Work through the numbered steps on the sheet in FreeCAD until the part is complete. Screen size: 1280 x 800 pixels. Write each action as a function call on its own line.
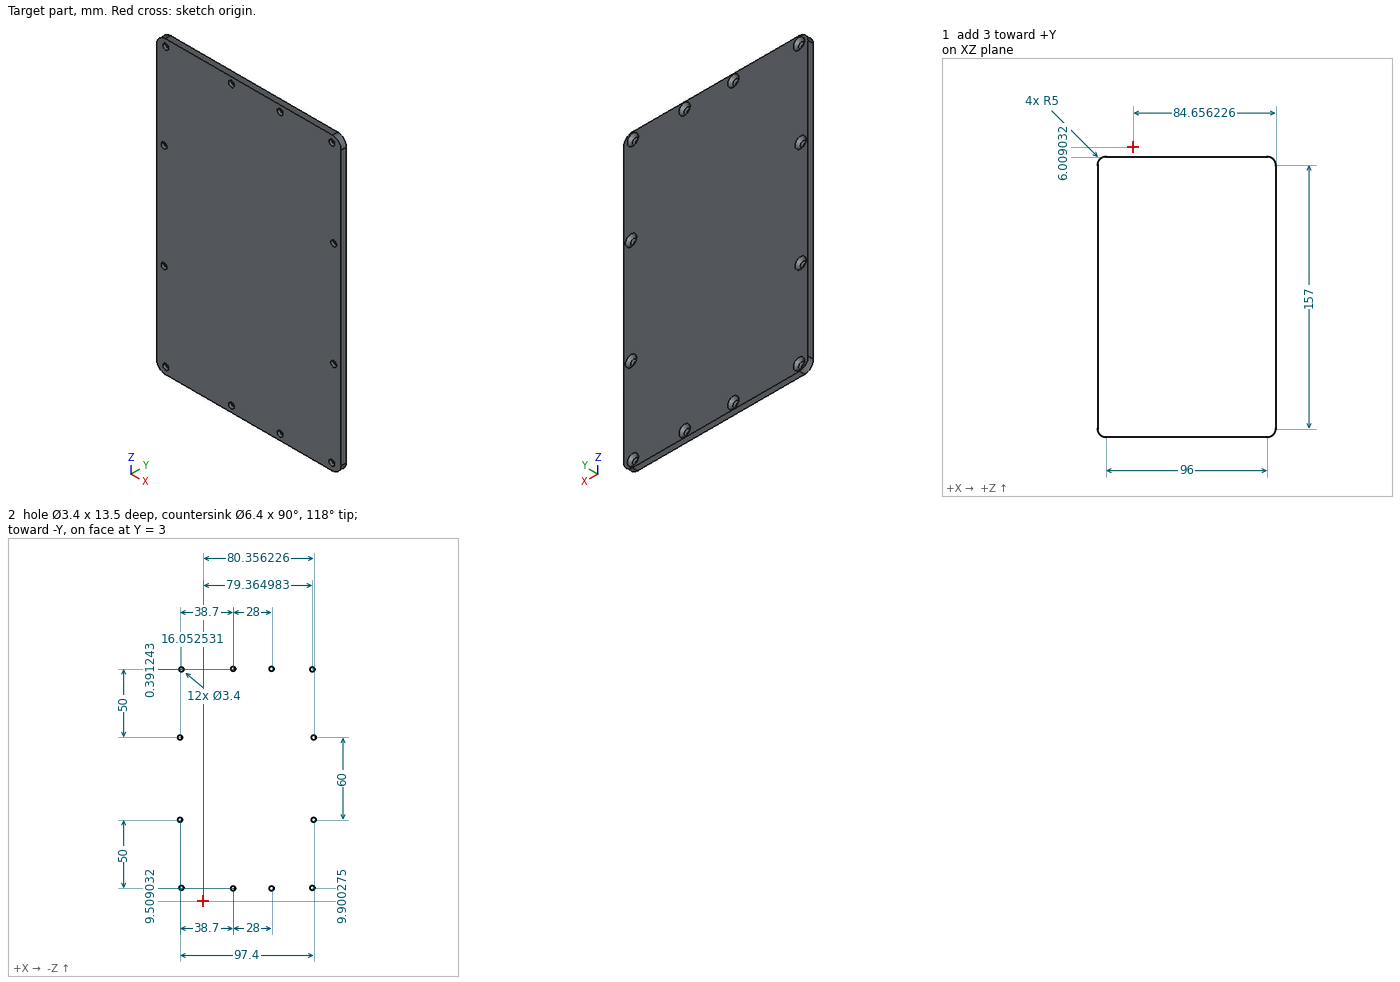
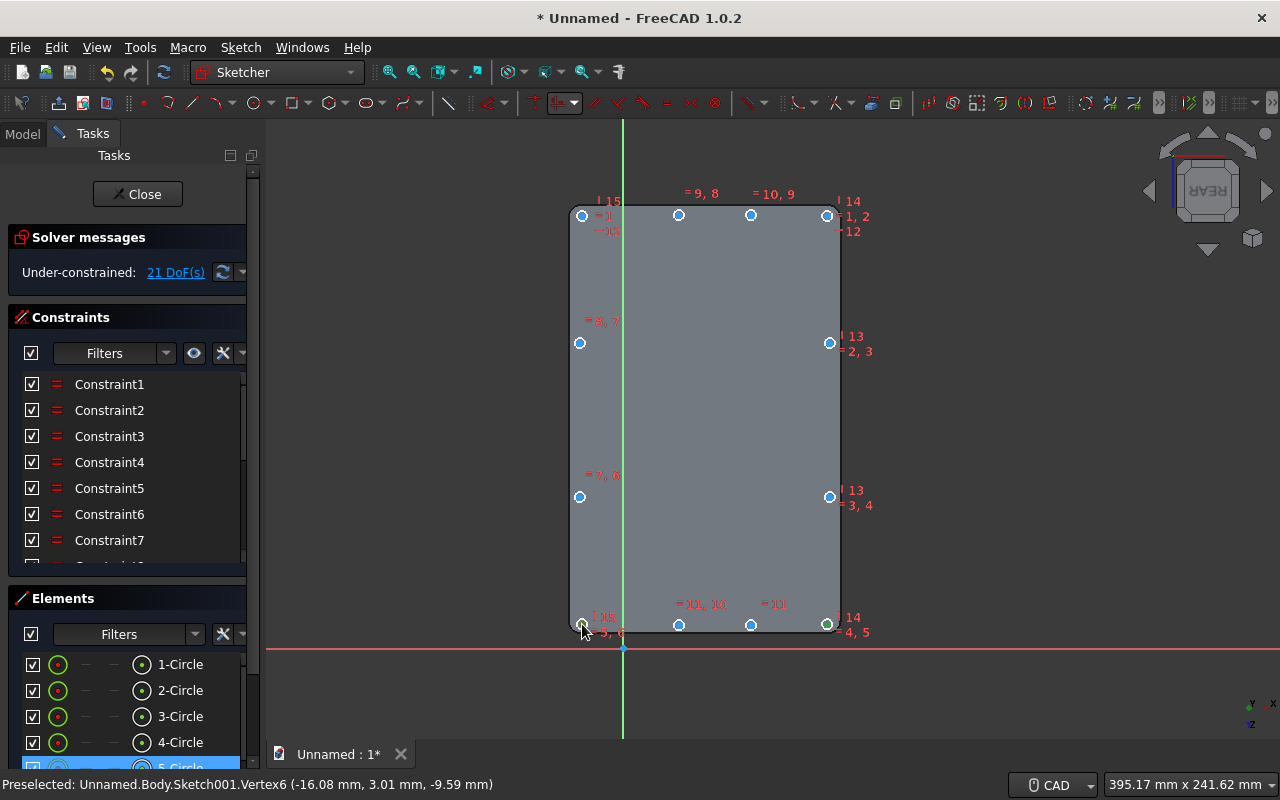
click(576, 104)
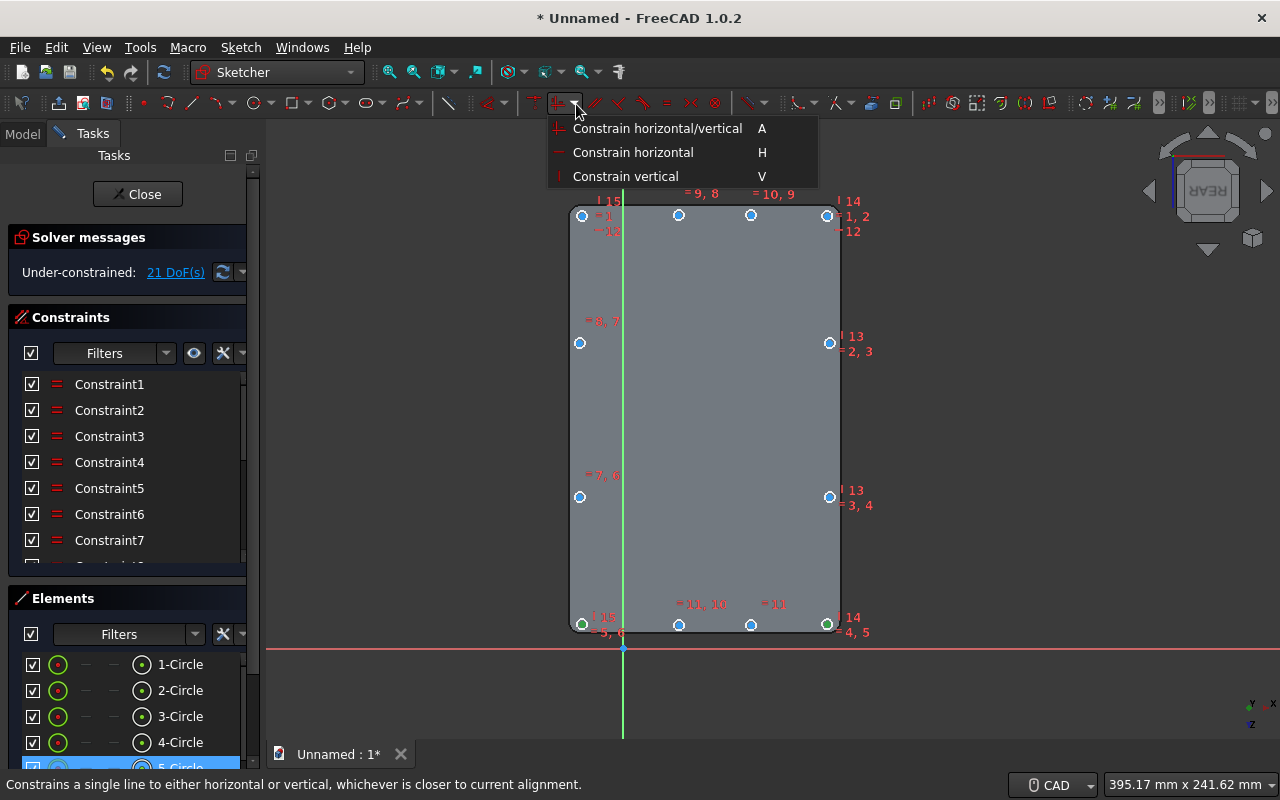
click(683, 152)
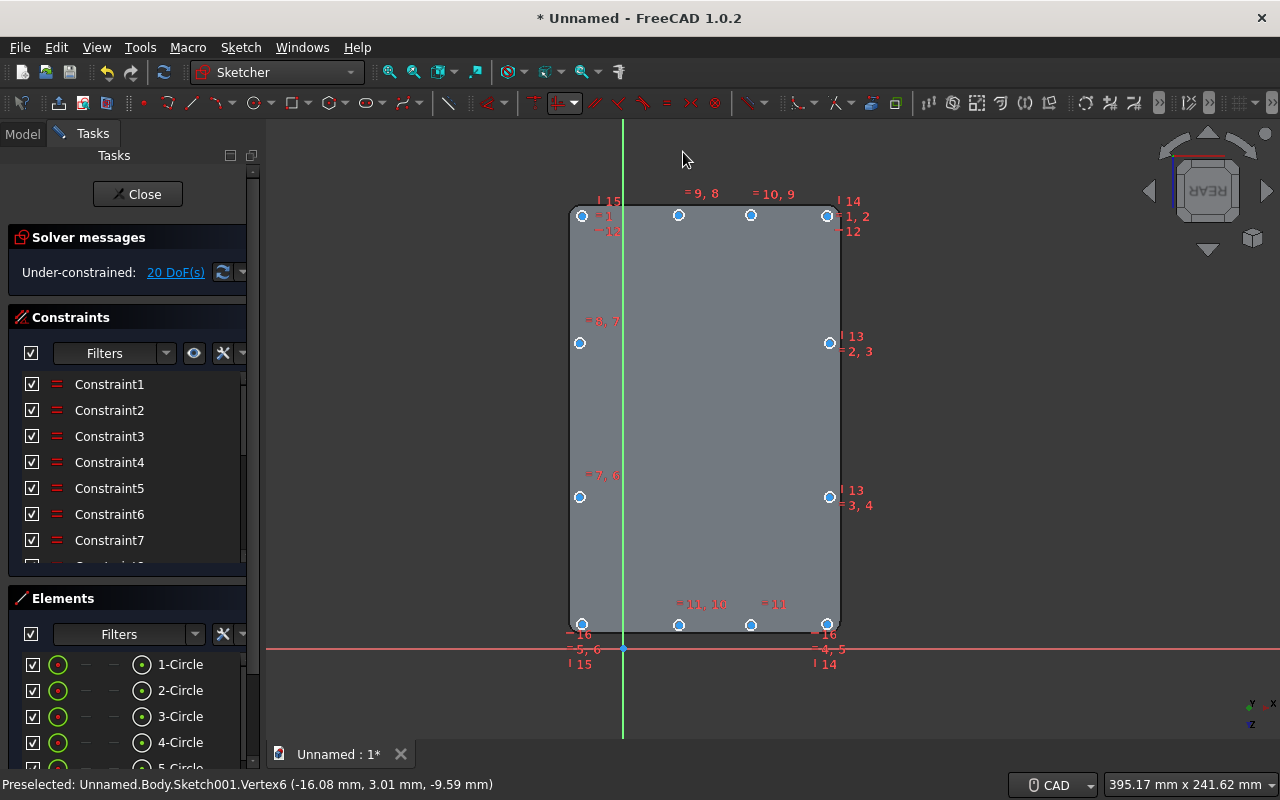
click(830, 497)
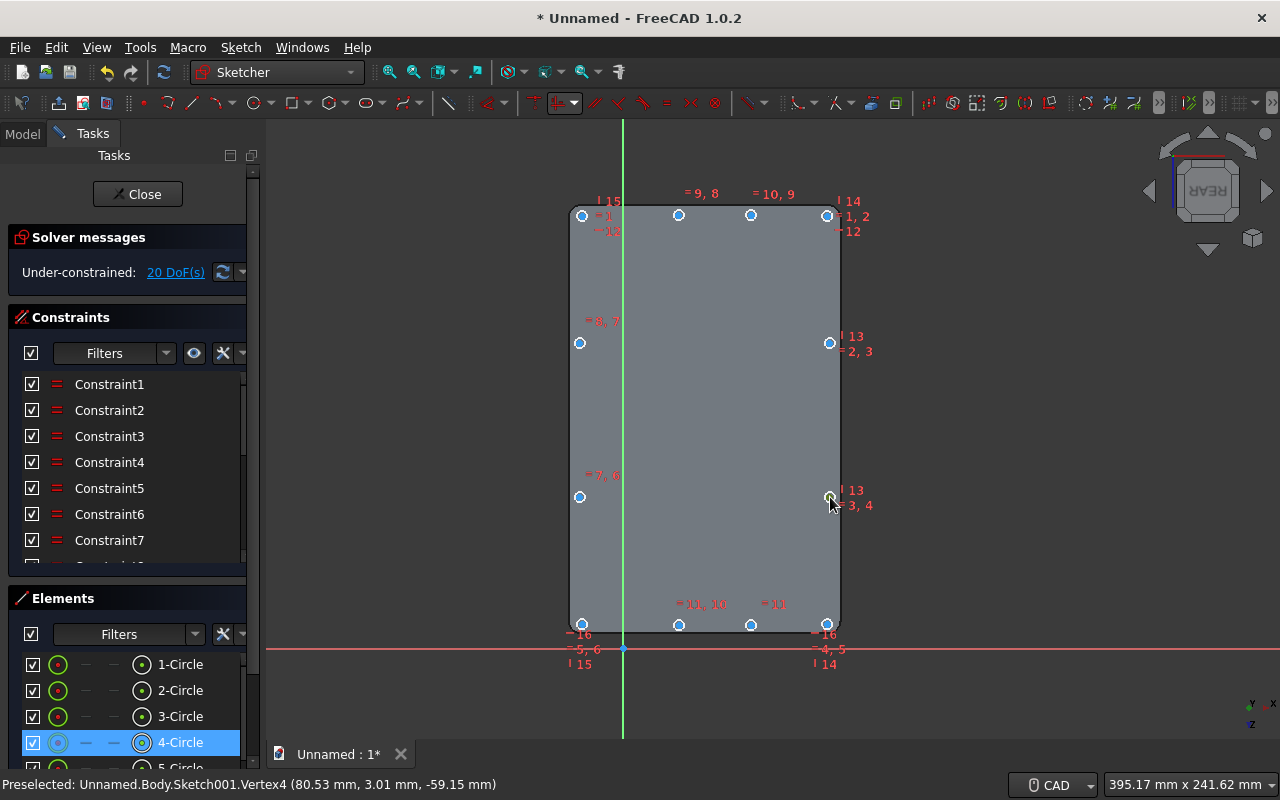
click(580, 497)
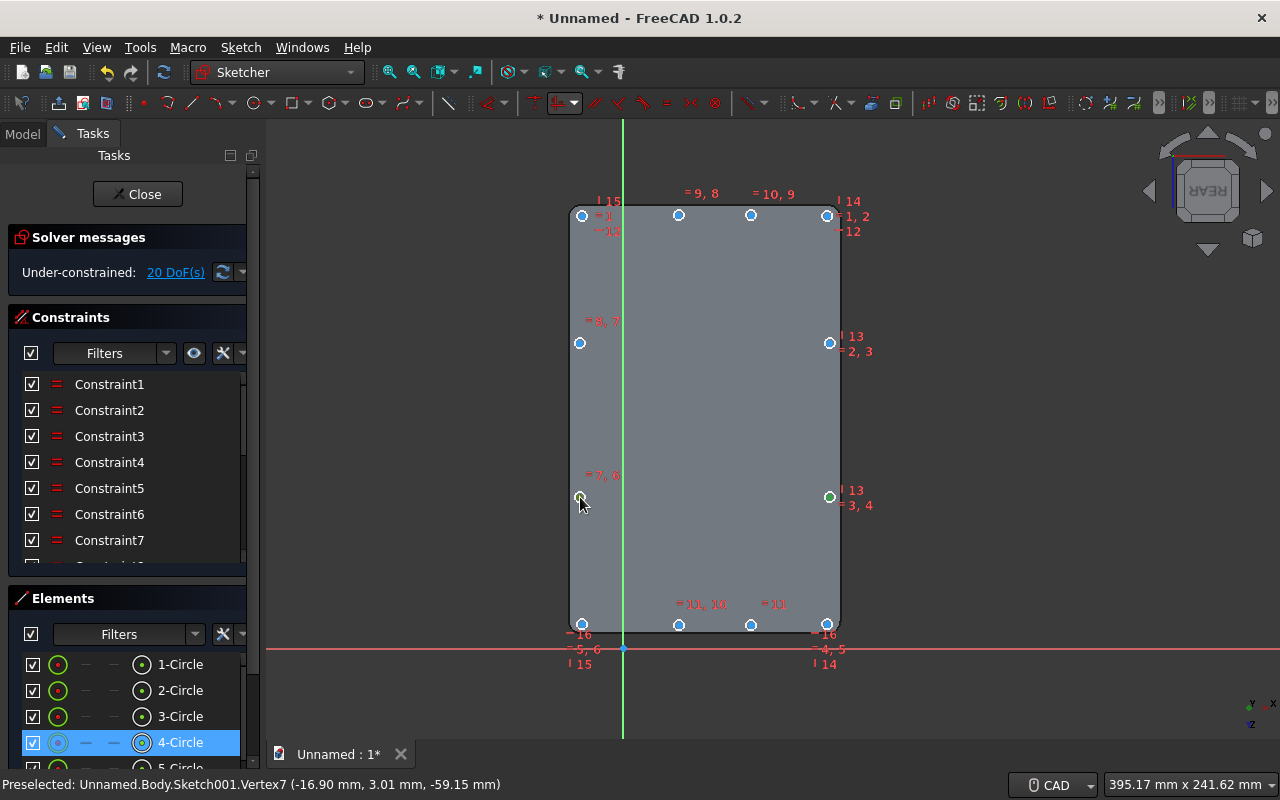
key(h)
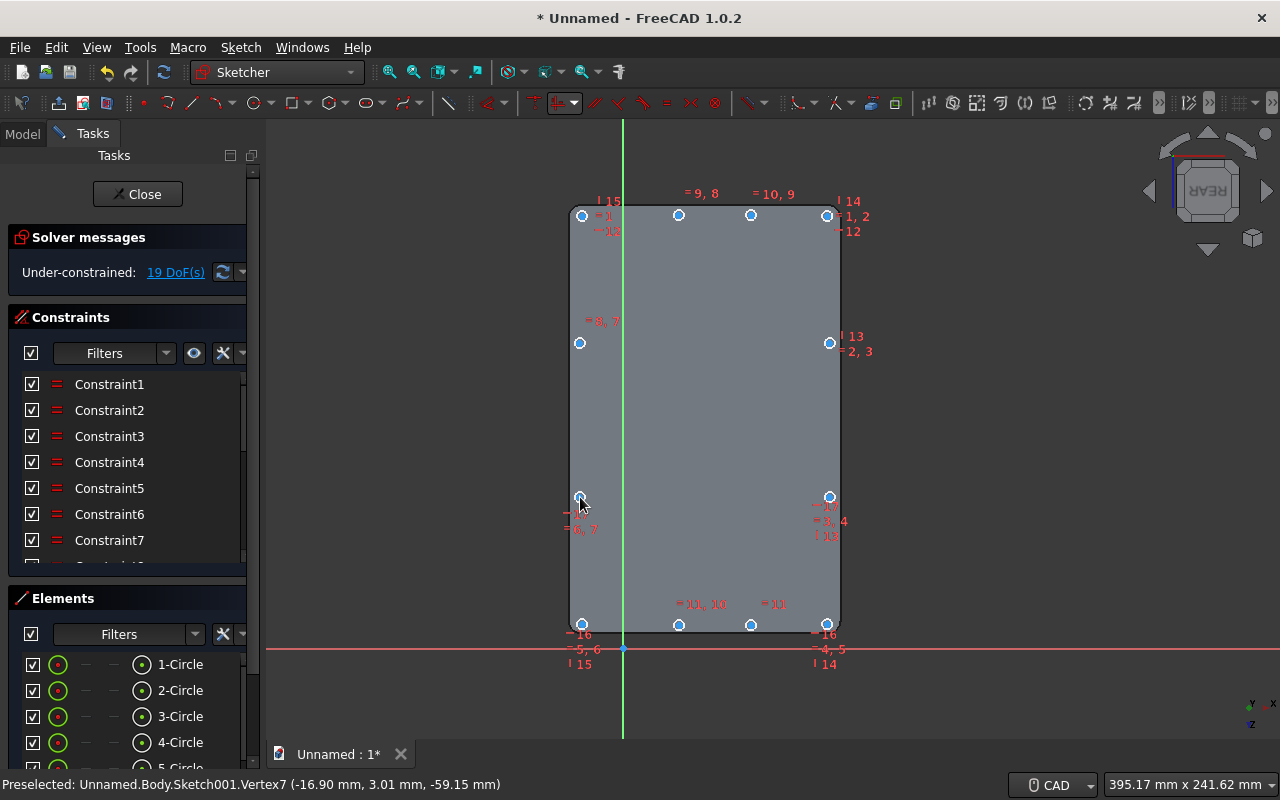
click(580, 497)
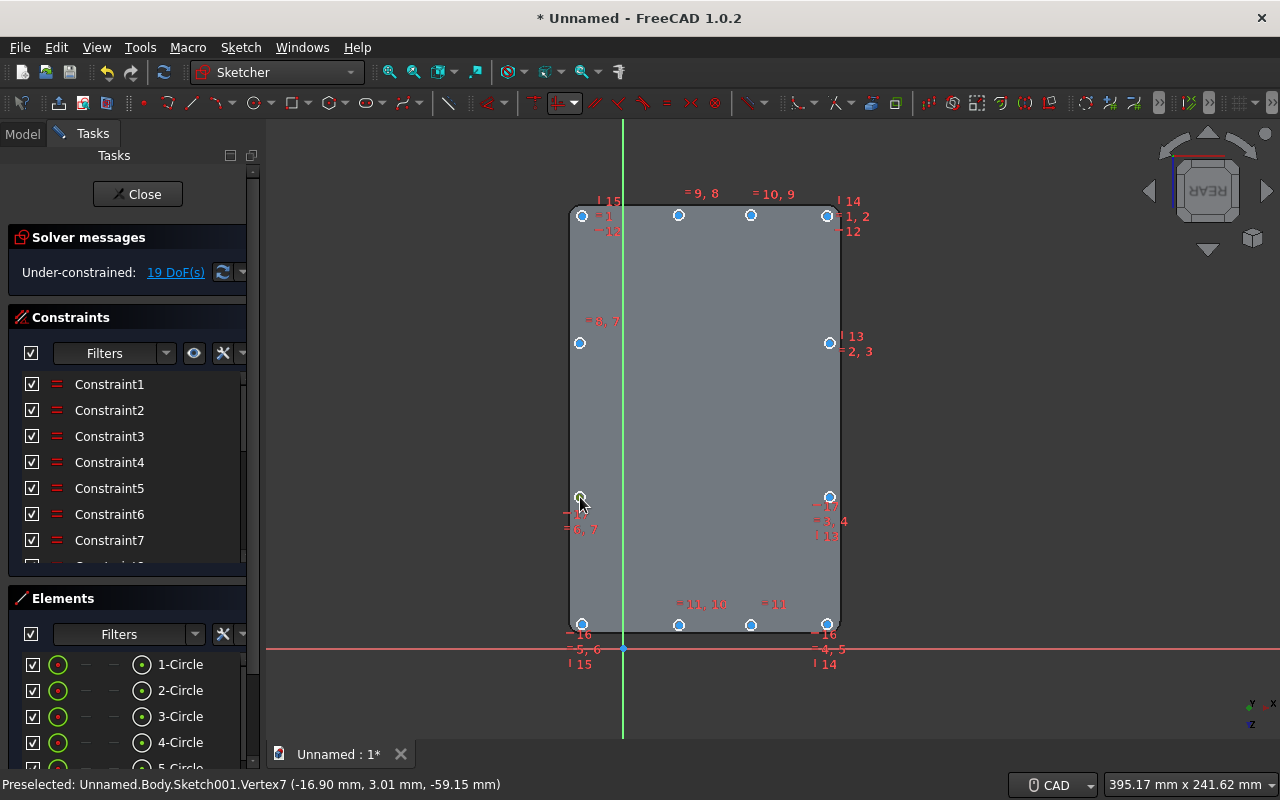
click(580, 343)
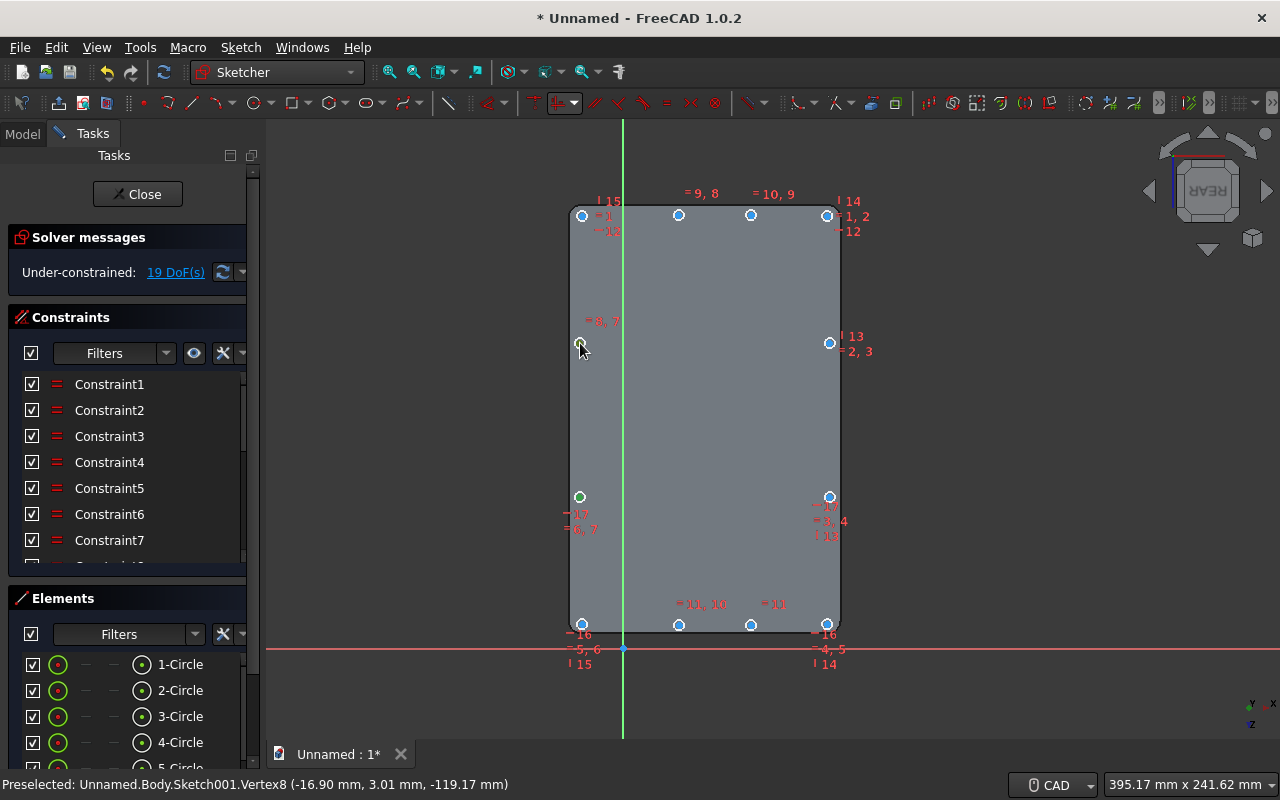
click(576, 104)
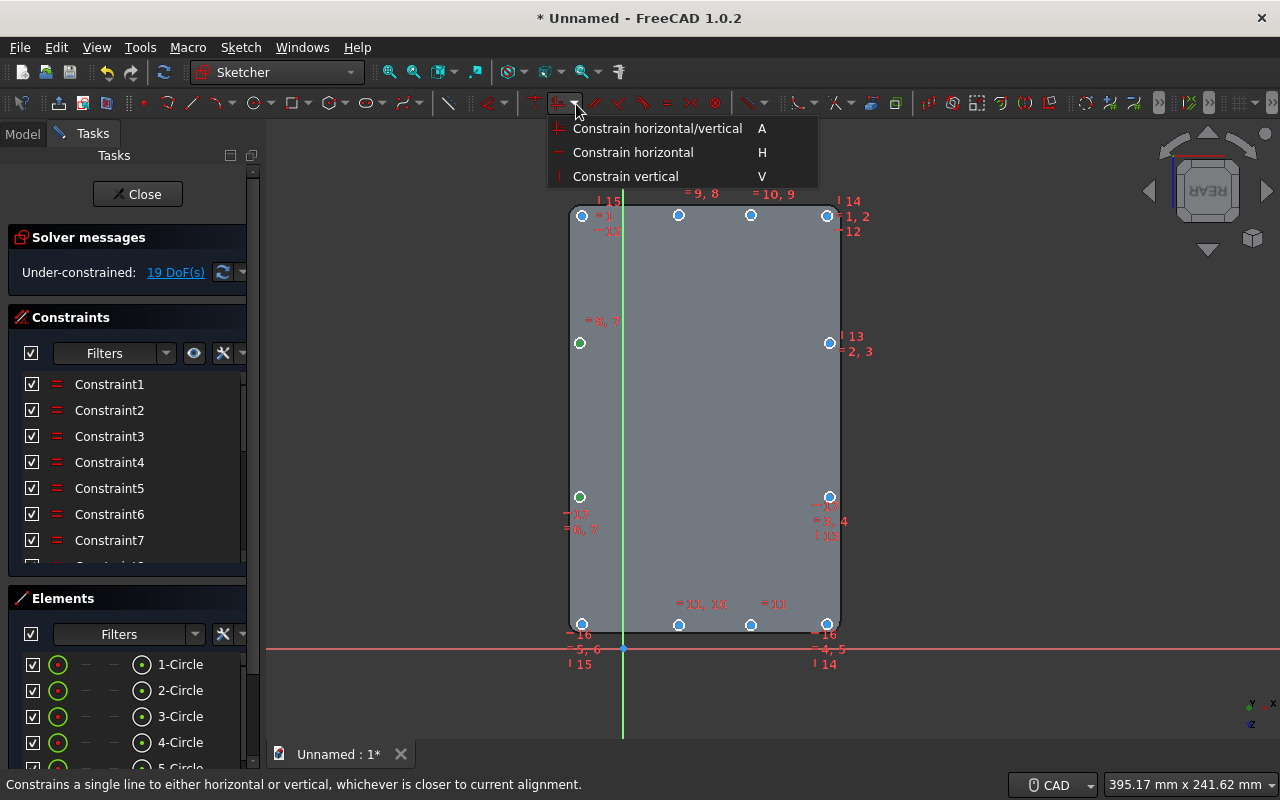
click(683, 176)